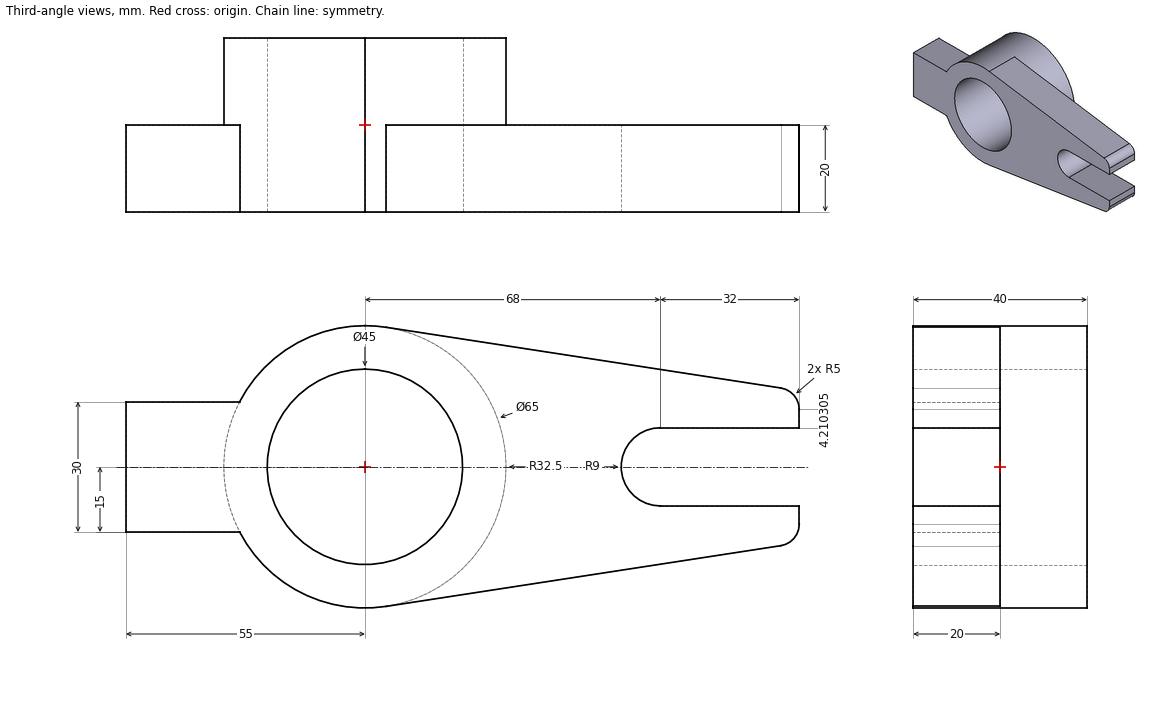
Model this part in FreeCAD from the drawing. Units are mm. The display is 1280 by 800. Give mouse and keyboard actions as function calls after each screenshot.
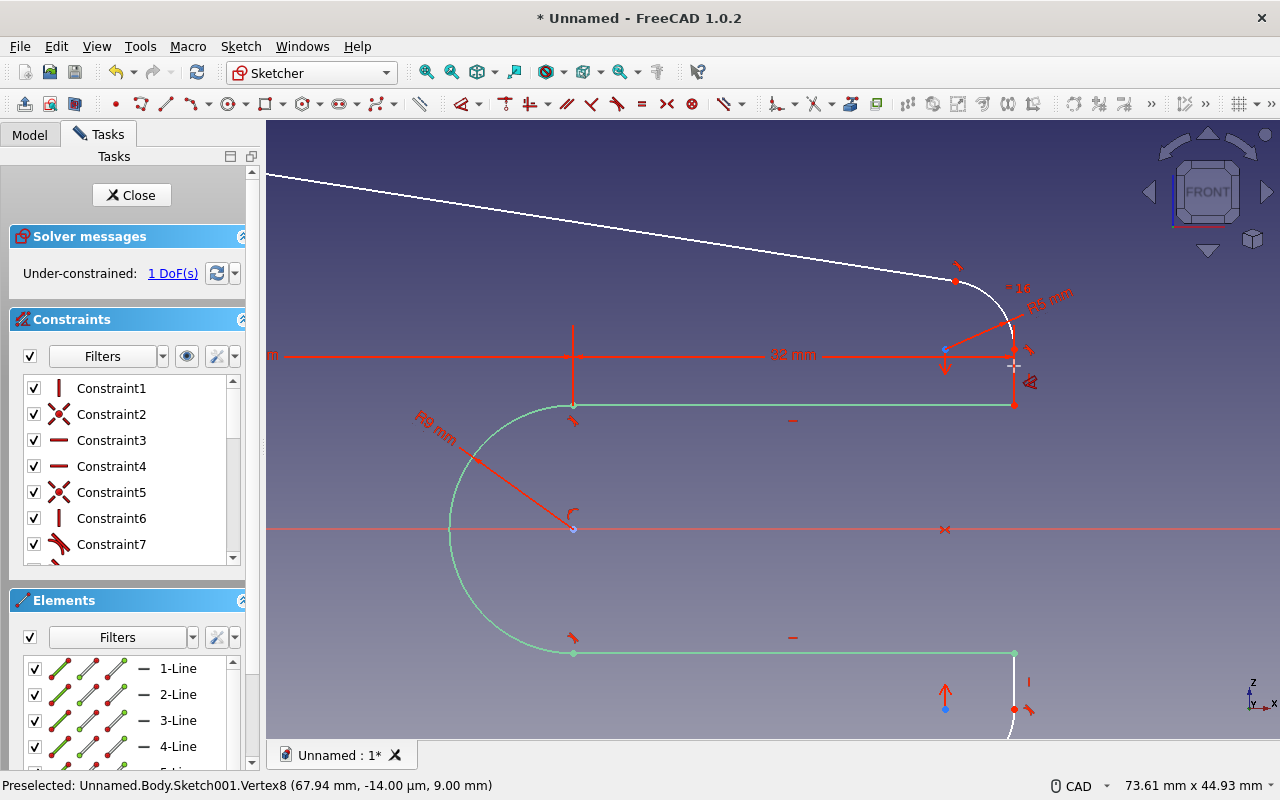
click(1014, 366)
click(1048, 377)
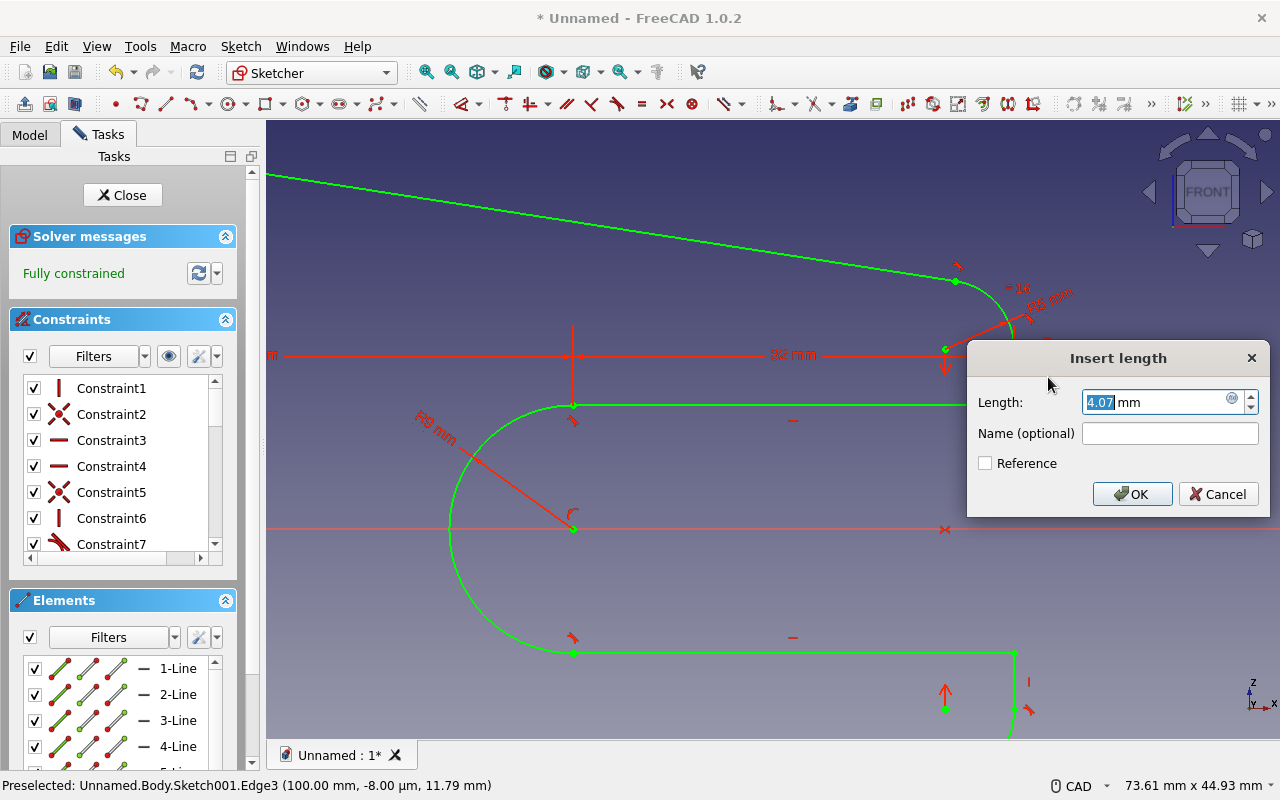
text(4.210305)
key(Return)
key(Escape)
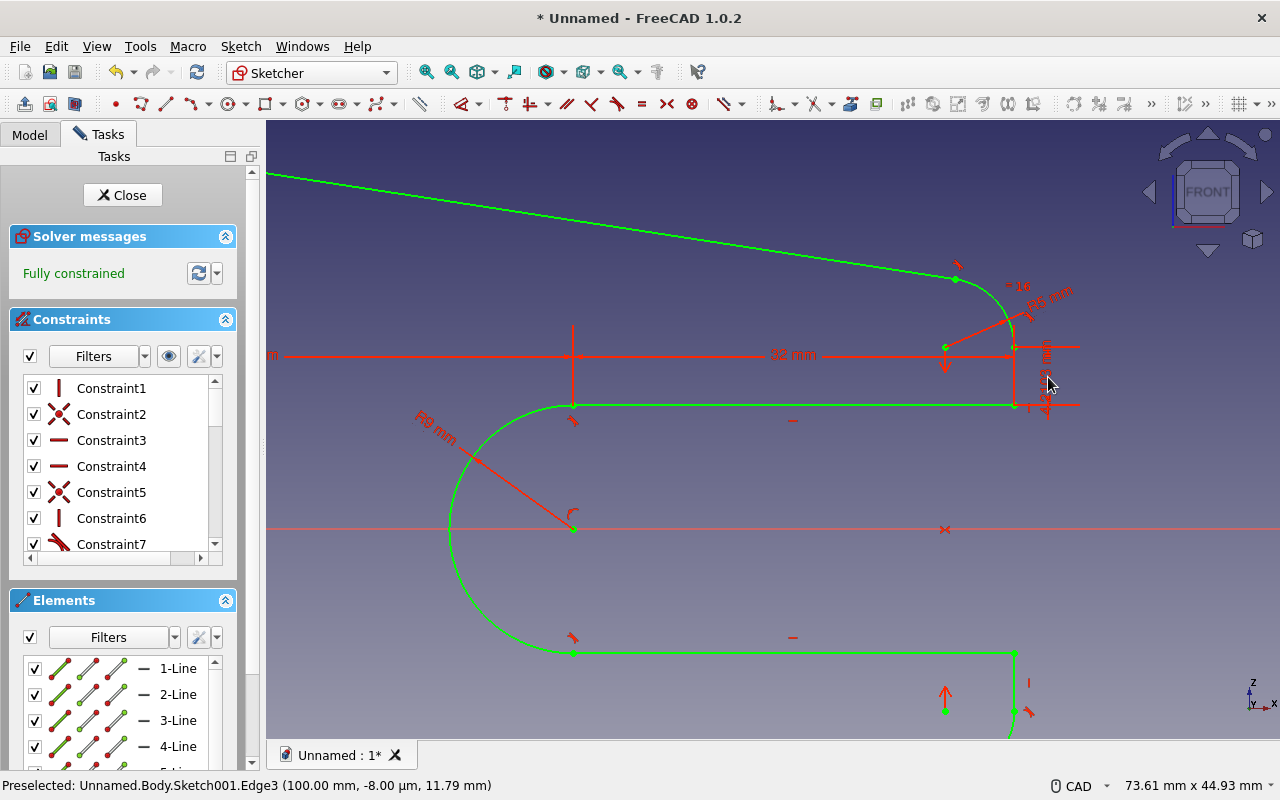
click(123, 195)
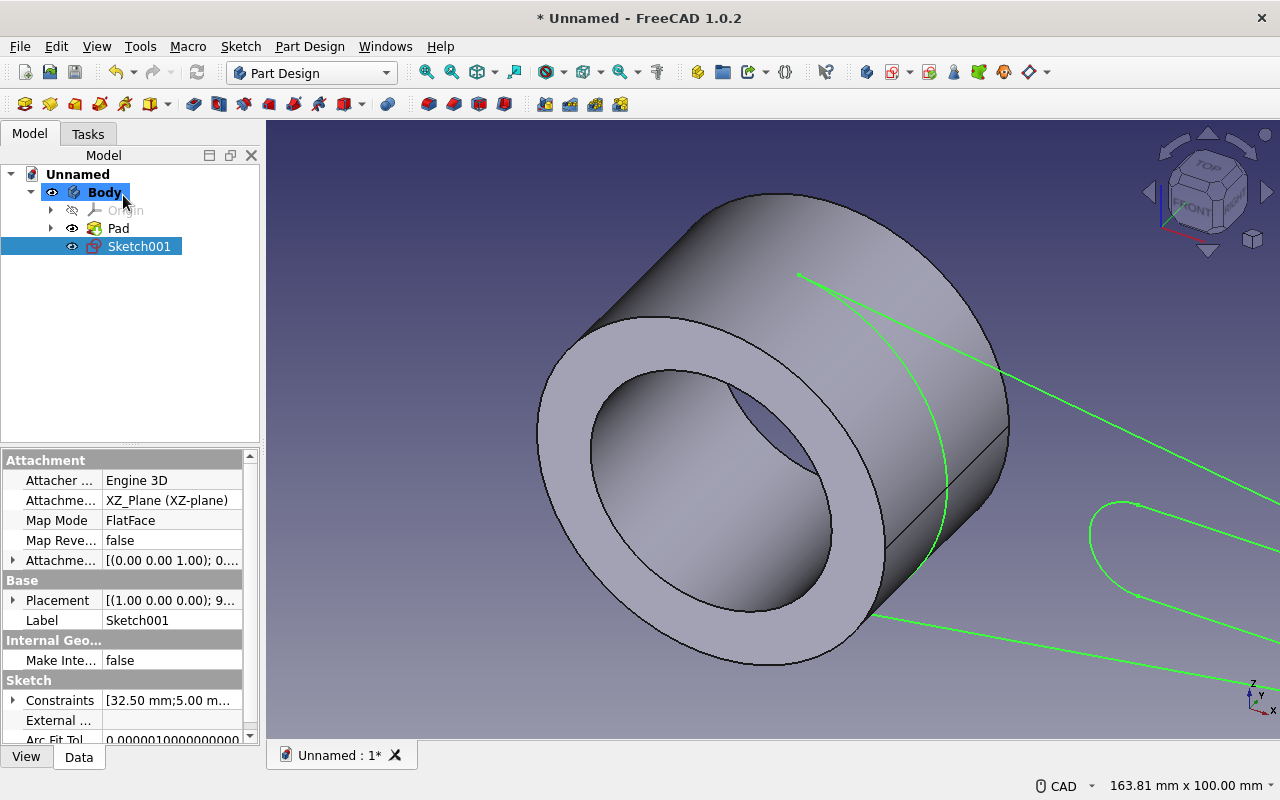
click(25, 104)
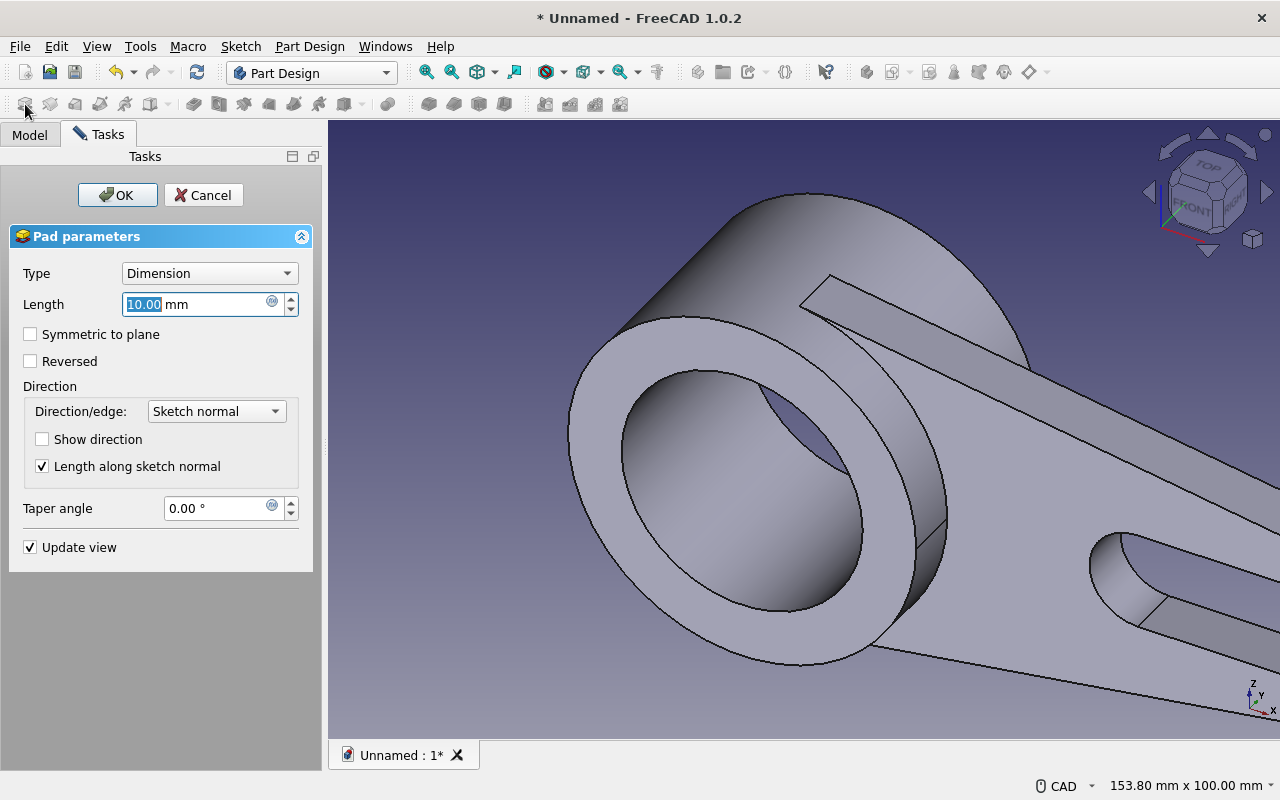
text(20)
key(Tab)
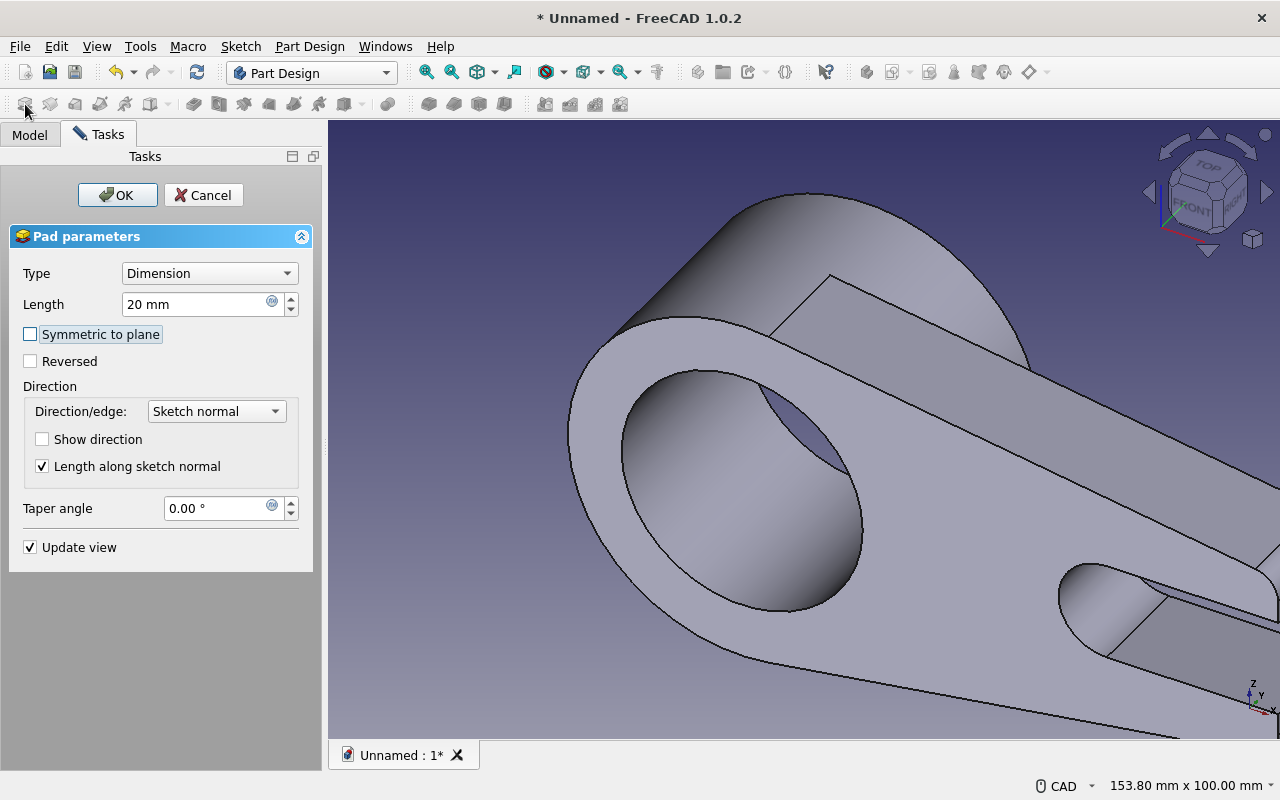
click(118, 195)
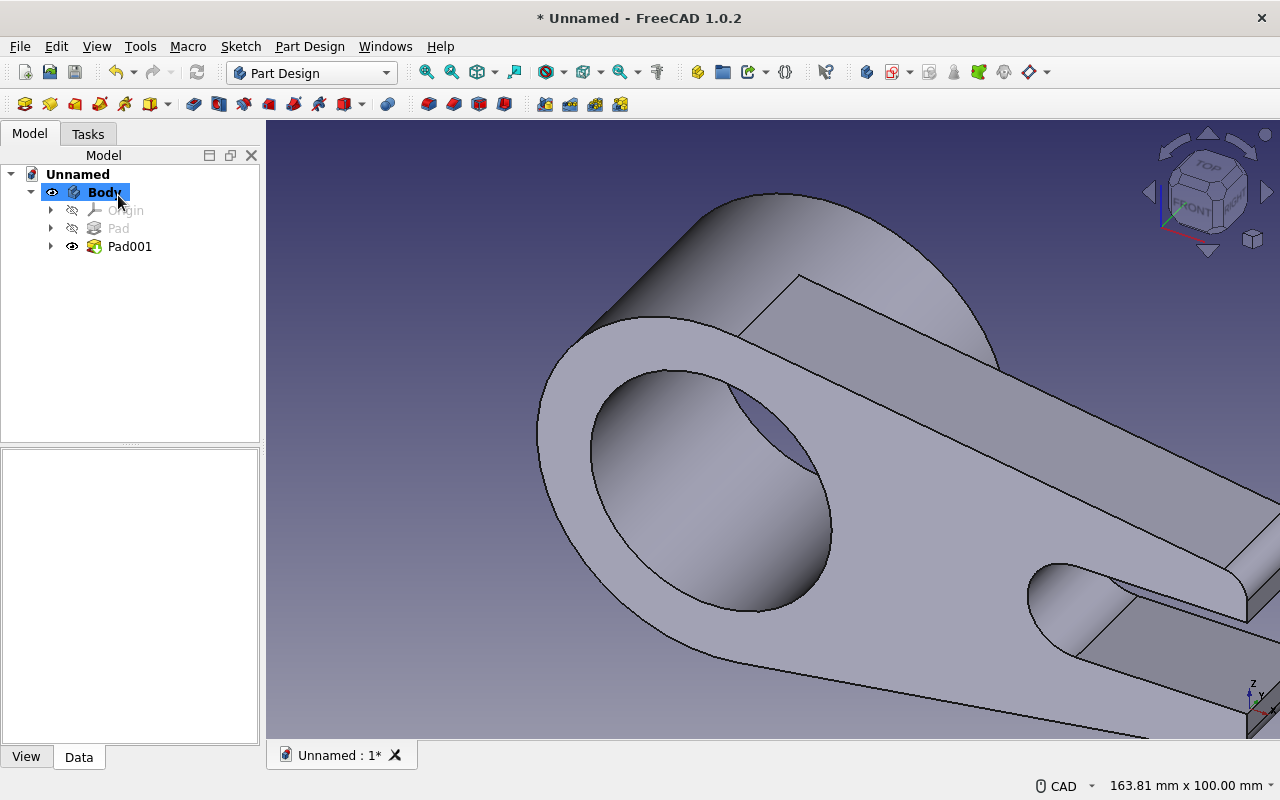
key(v)
key(f)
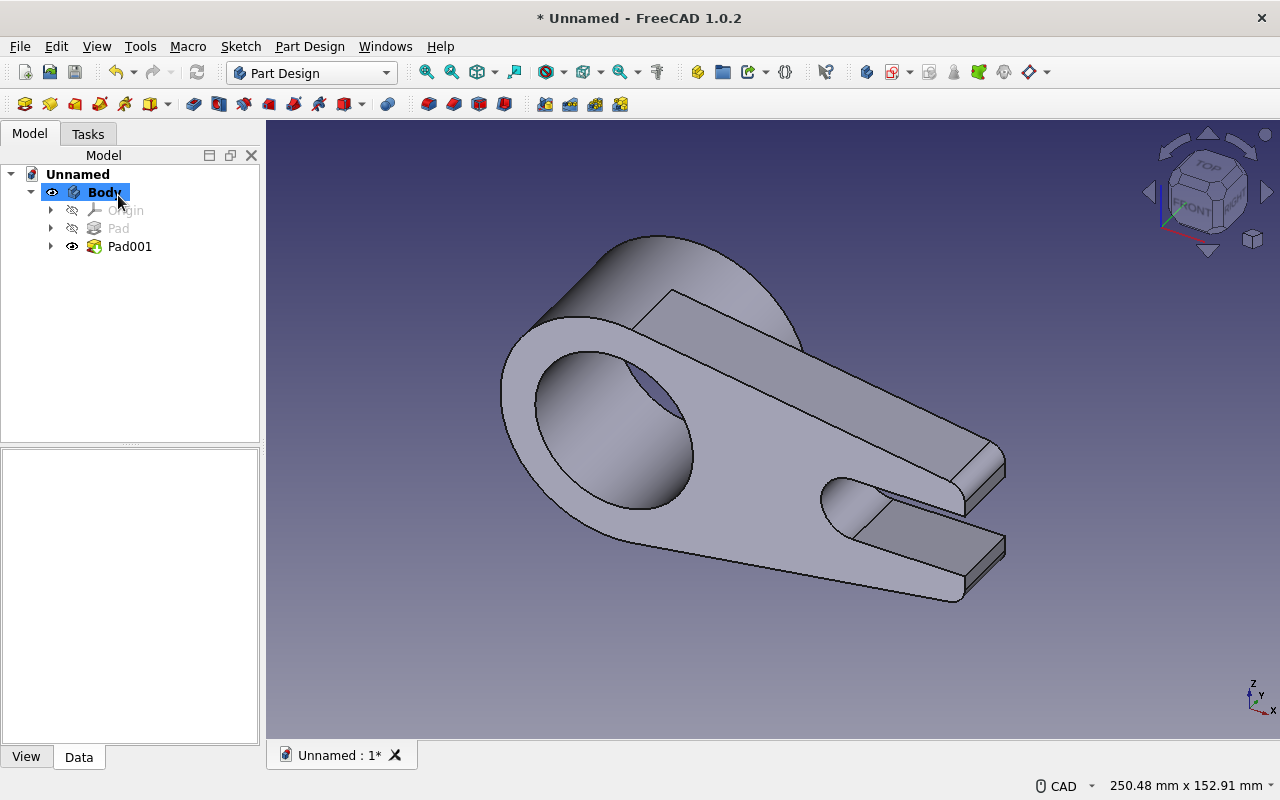
key(4)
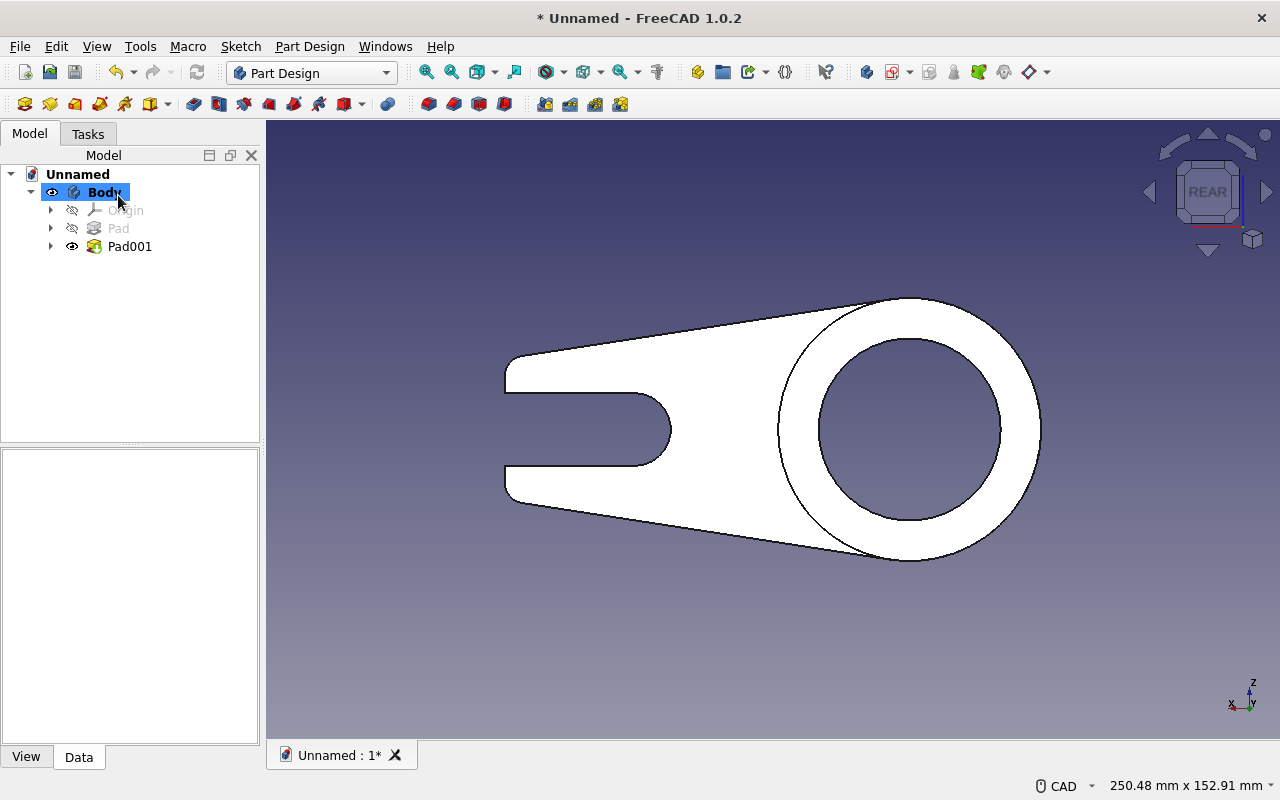
click(697, 391)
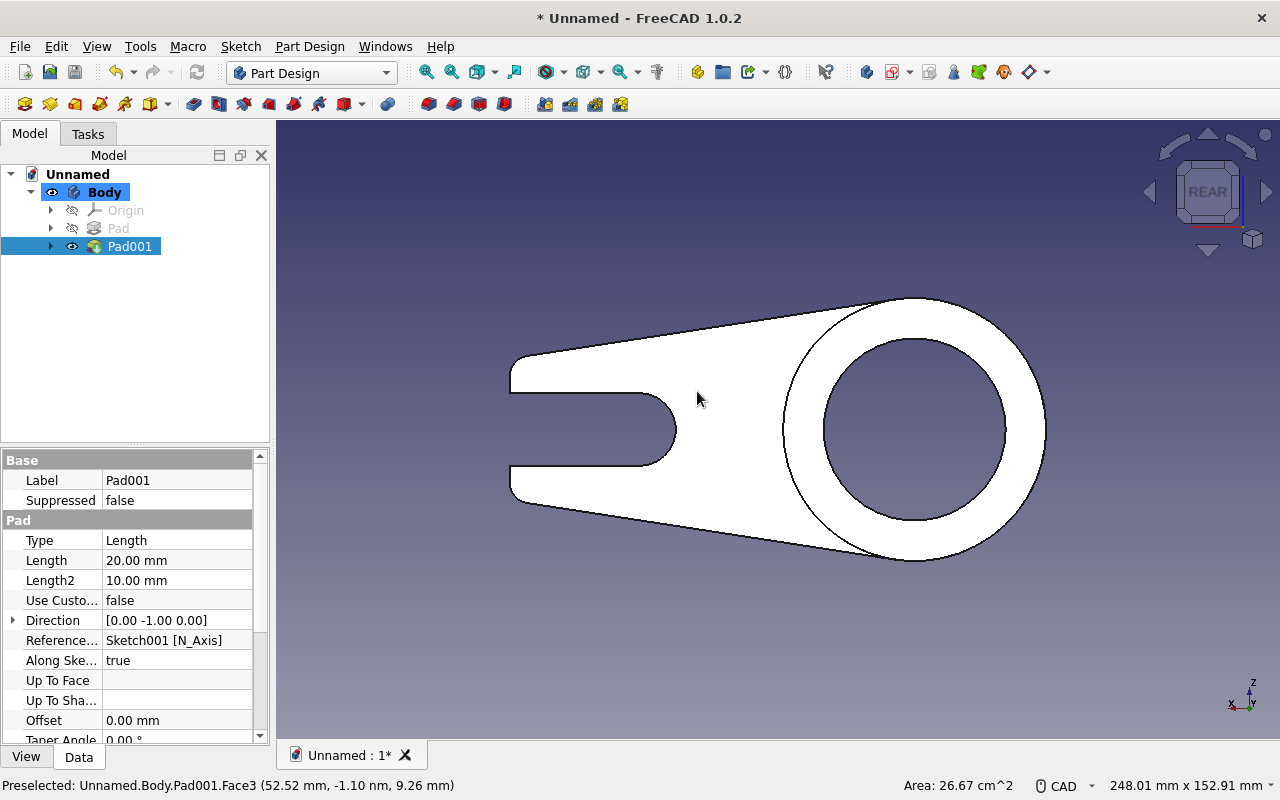
click(892, 72)